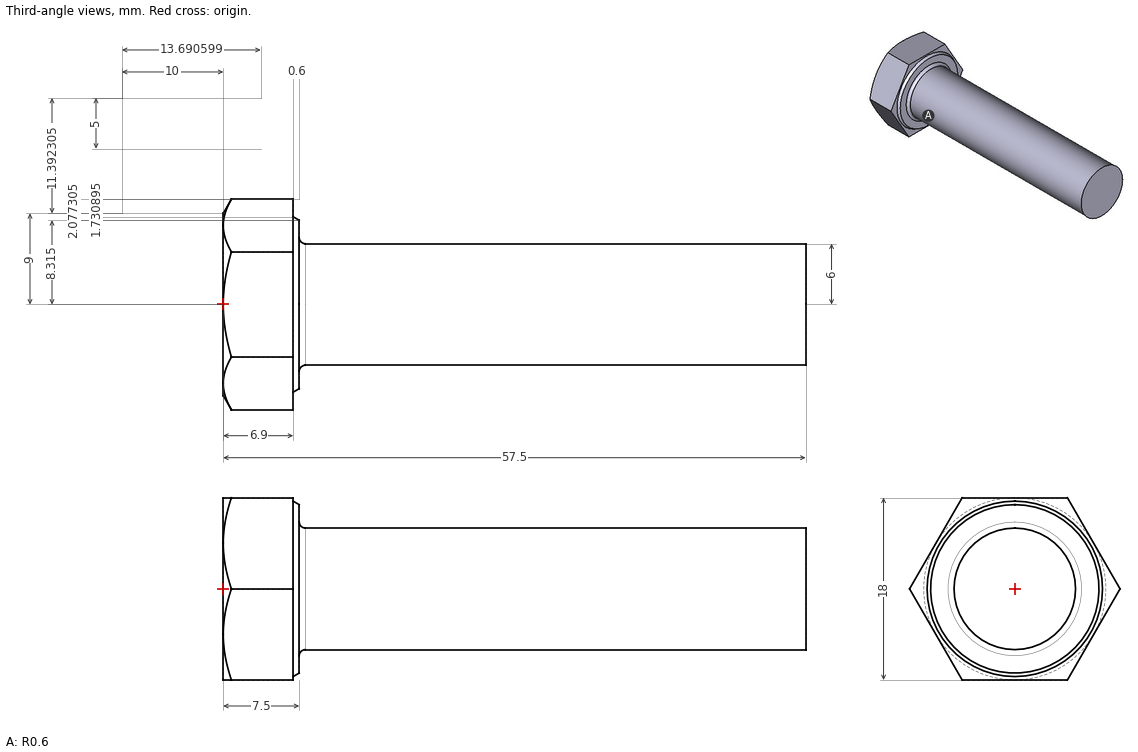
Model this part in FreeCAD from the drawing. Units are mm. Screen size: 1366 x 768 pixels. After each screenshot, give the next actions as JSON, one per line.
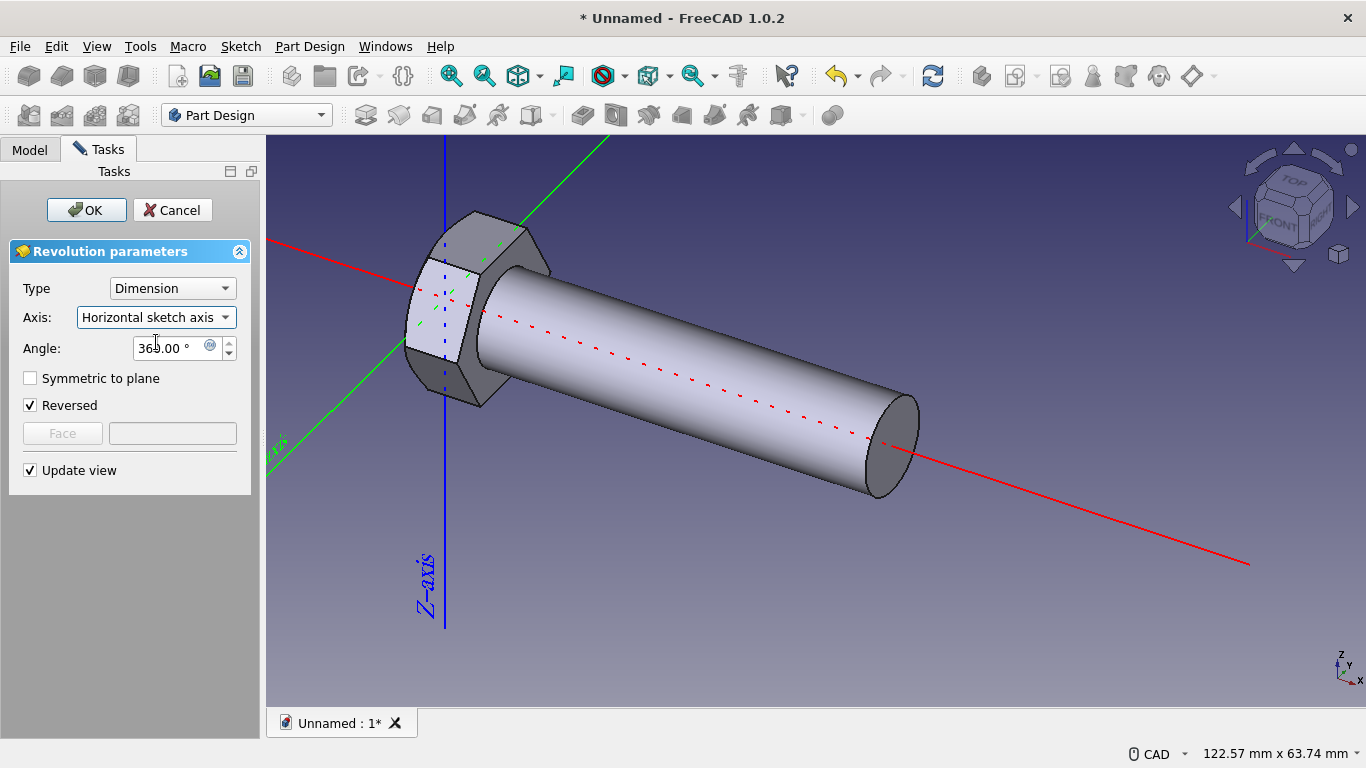
{"action": "left_click", "coordinate": [87, 210]}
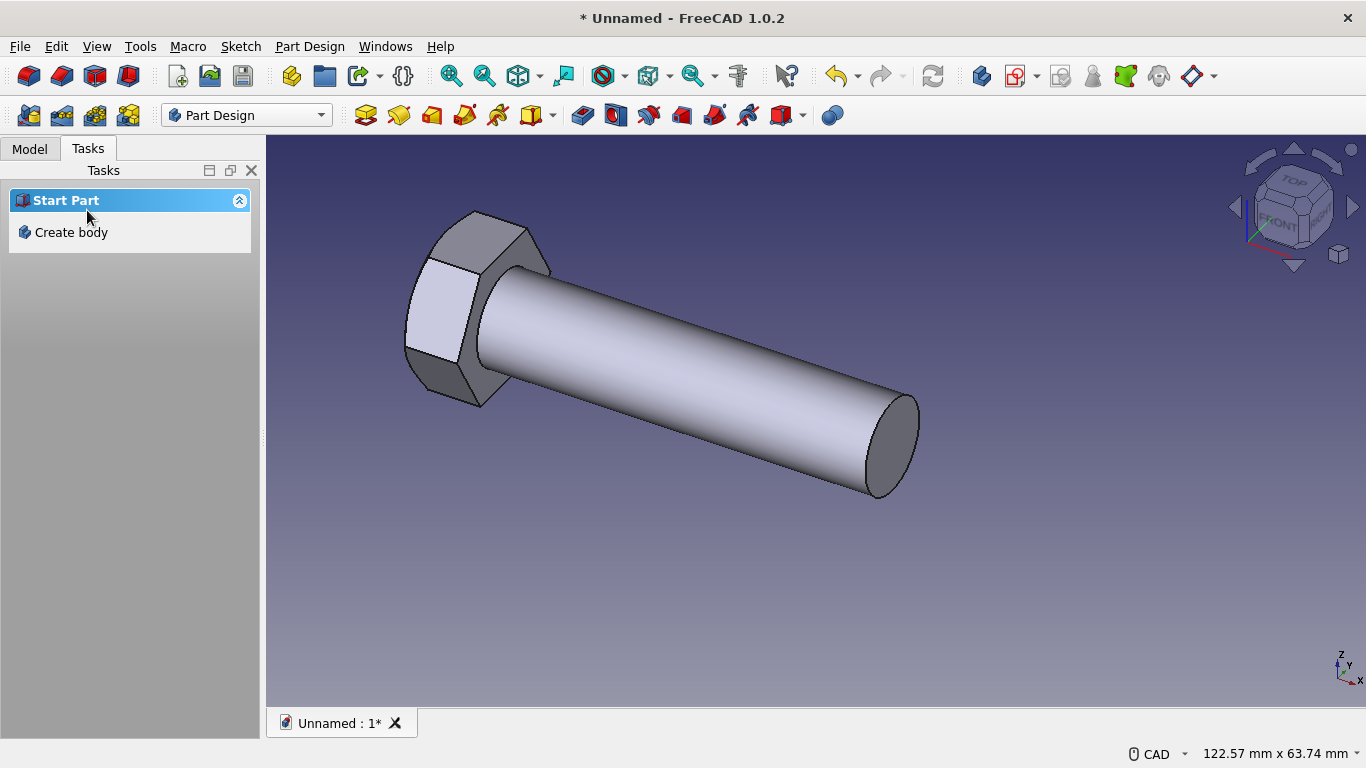
{"action": "left_click", "coordinate": [1014, 76]}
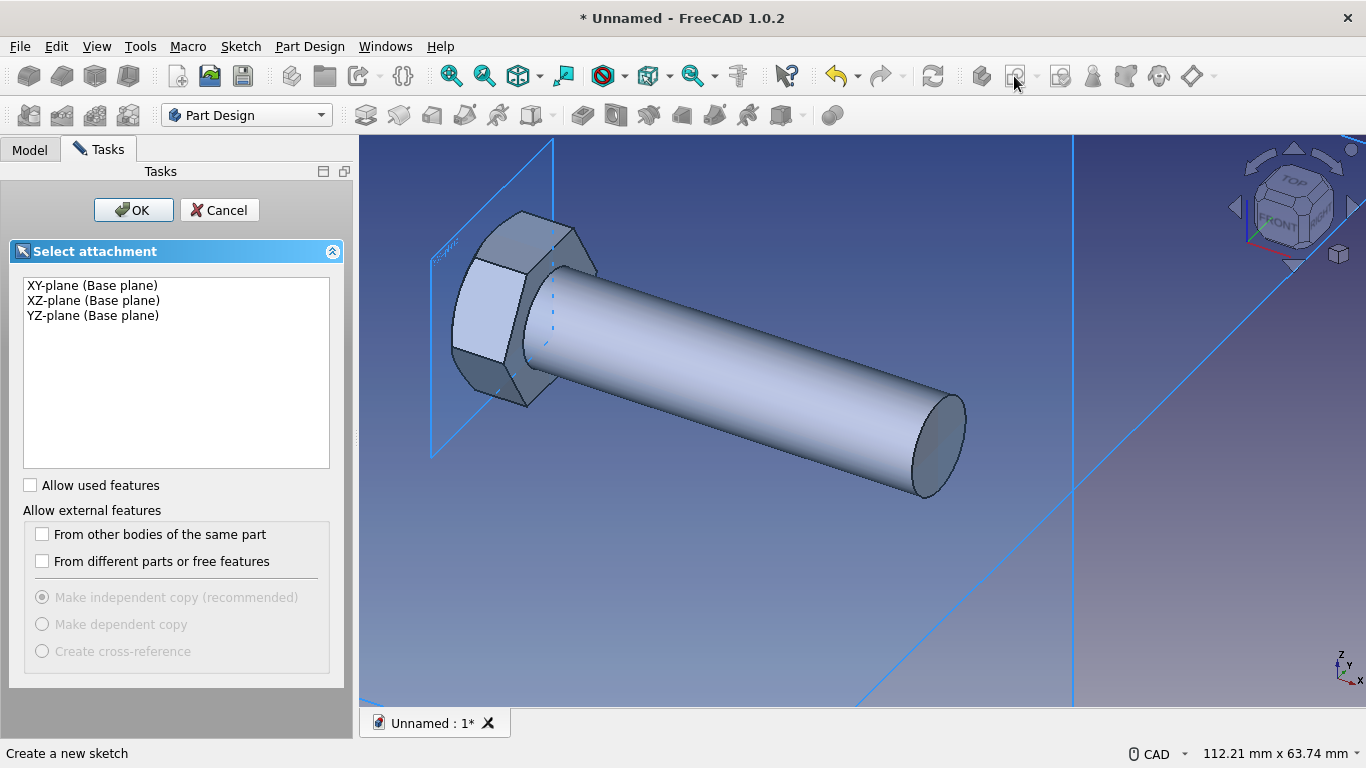
{"action": "left_click", "coordinate": [84, 286]}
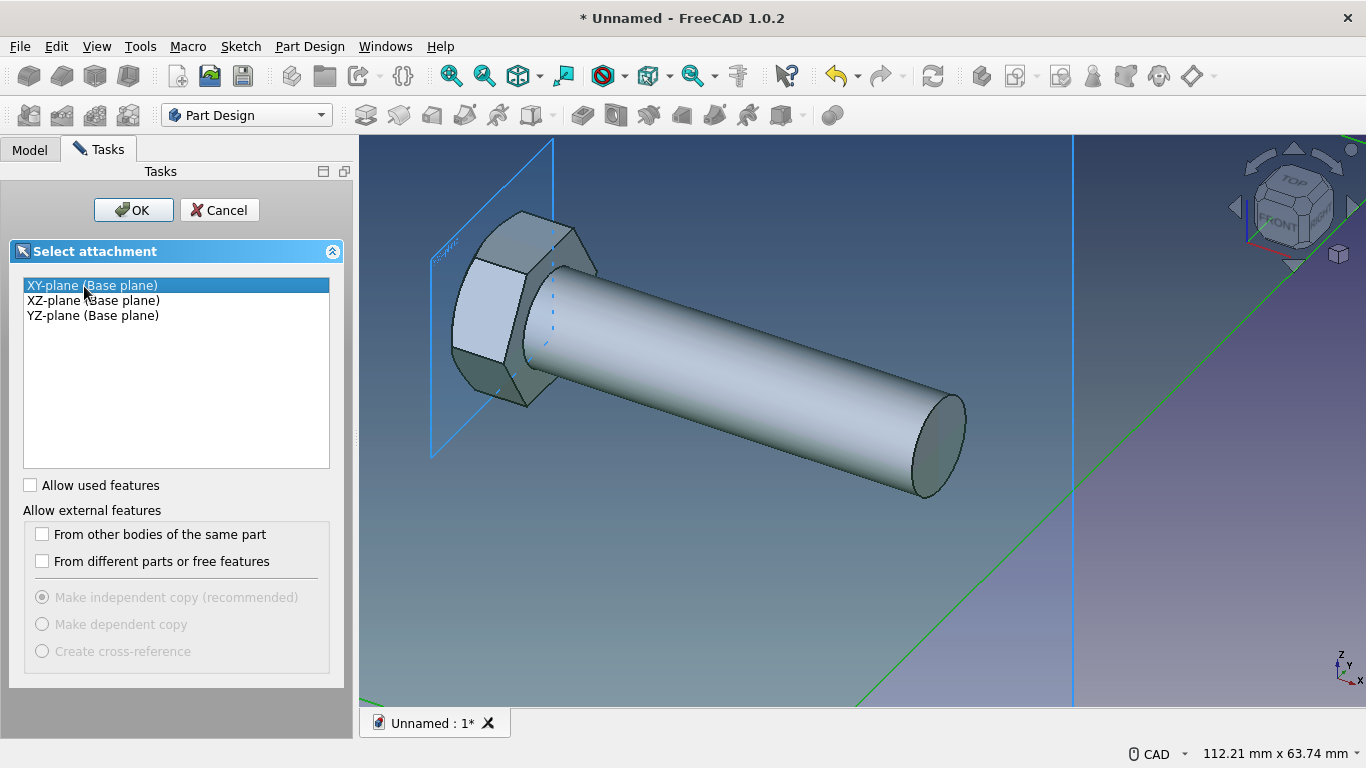
{"action": "left_click", "coordinate": [134, 210]}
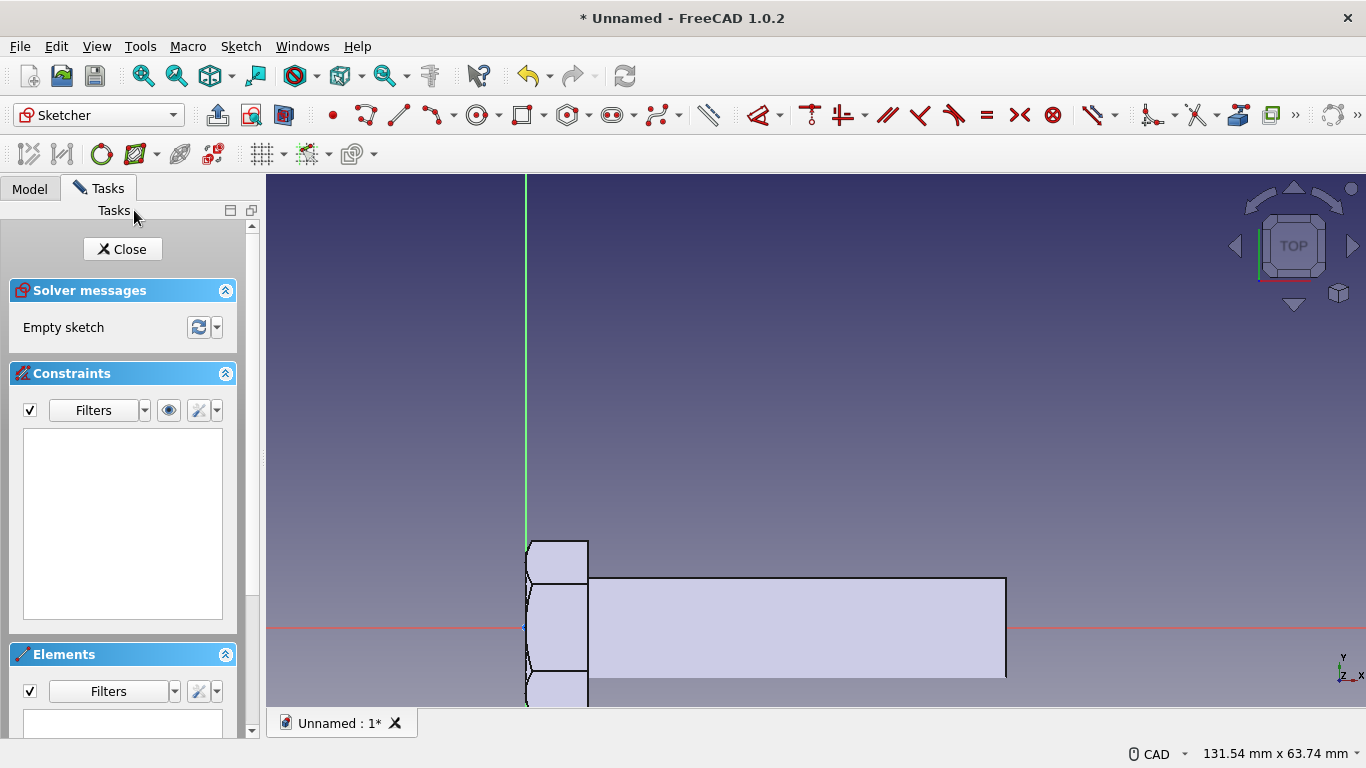
{"action": "key", "text": "q s"}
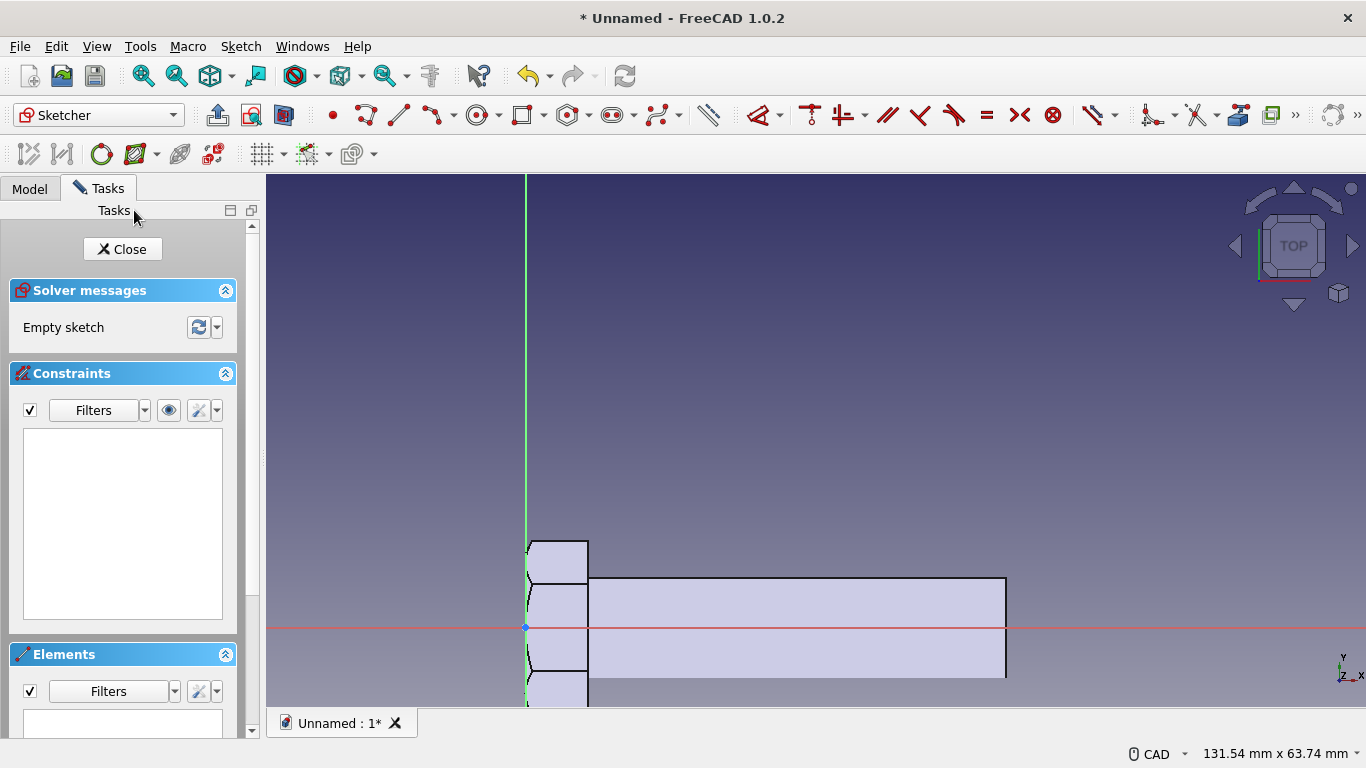
{"action": "scroll", "coordinate": [577, 555], "scroll_direction": "up", "scroll_amount": 15}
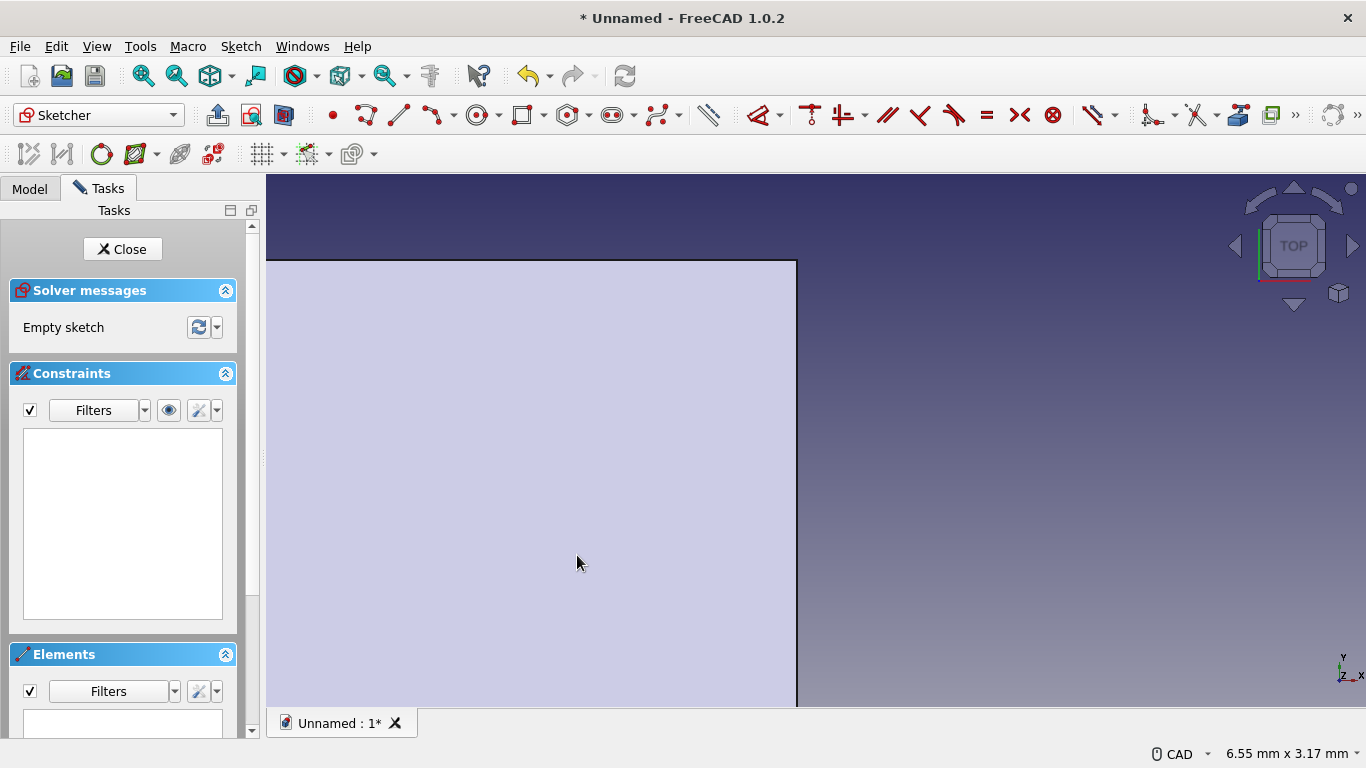
{"action": "key", "text": "g m"}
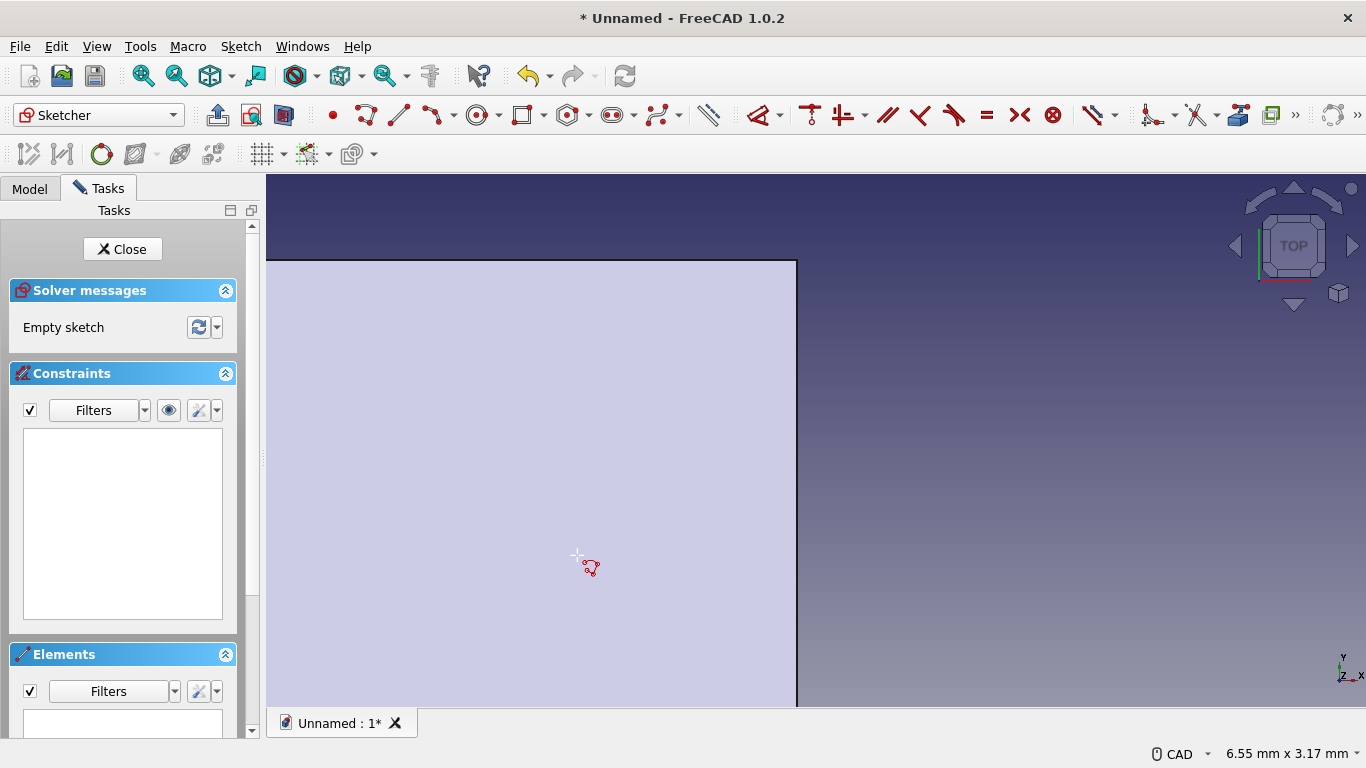
{"action": "left_click", "coordinate": [696, 551]}
{"action": "left_click", "coordinate": [797, 609]}
{"action": "left_click", "coordinate": [797, 260]}
{"action": "left_click", "coordinate": [696, 260]}
{"action": "left_click", "coordinate": [696, 552]}
{"action": "key", "text": "Escape"}
{"action": "key", "text": "Escape"}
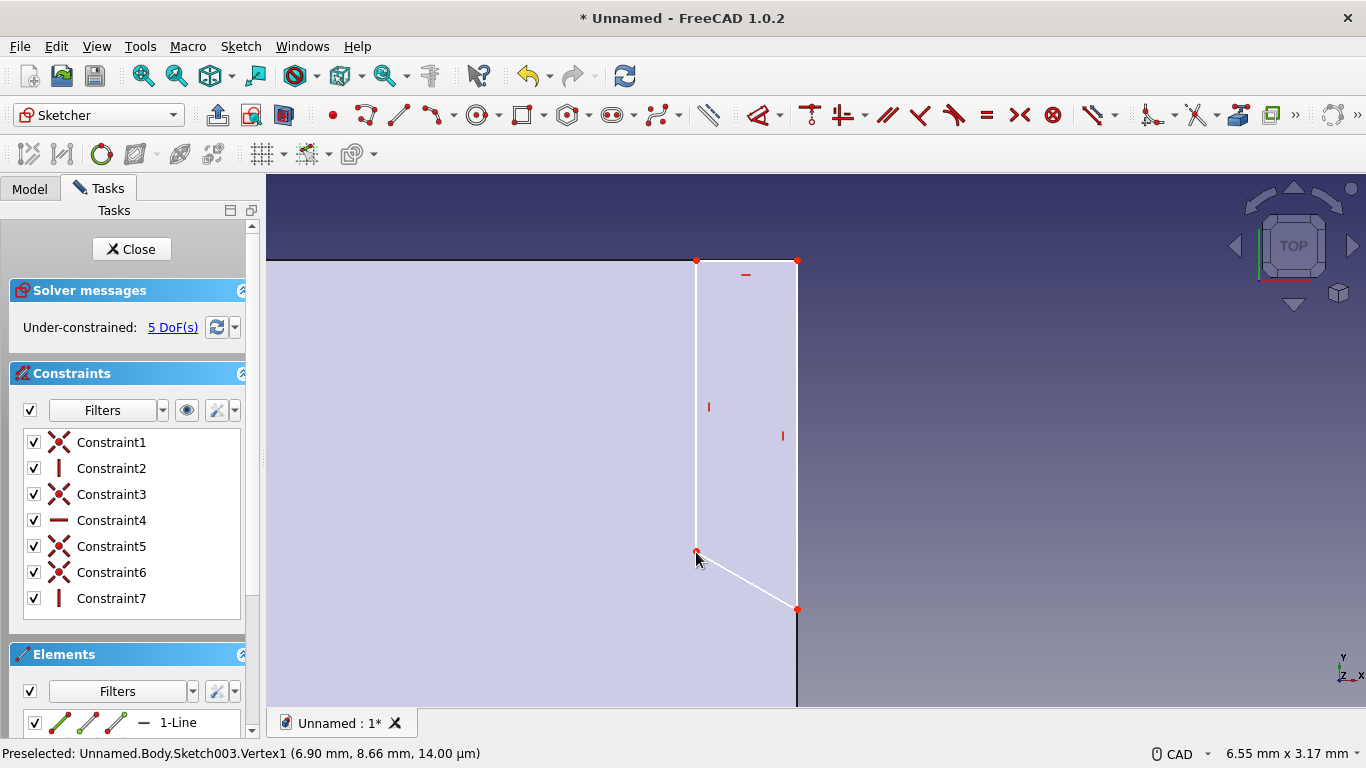
{"action": "left_click", "coordinate": [758, 116]}